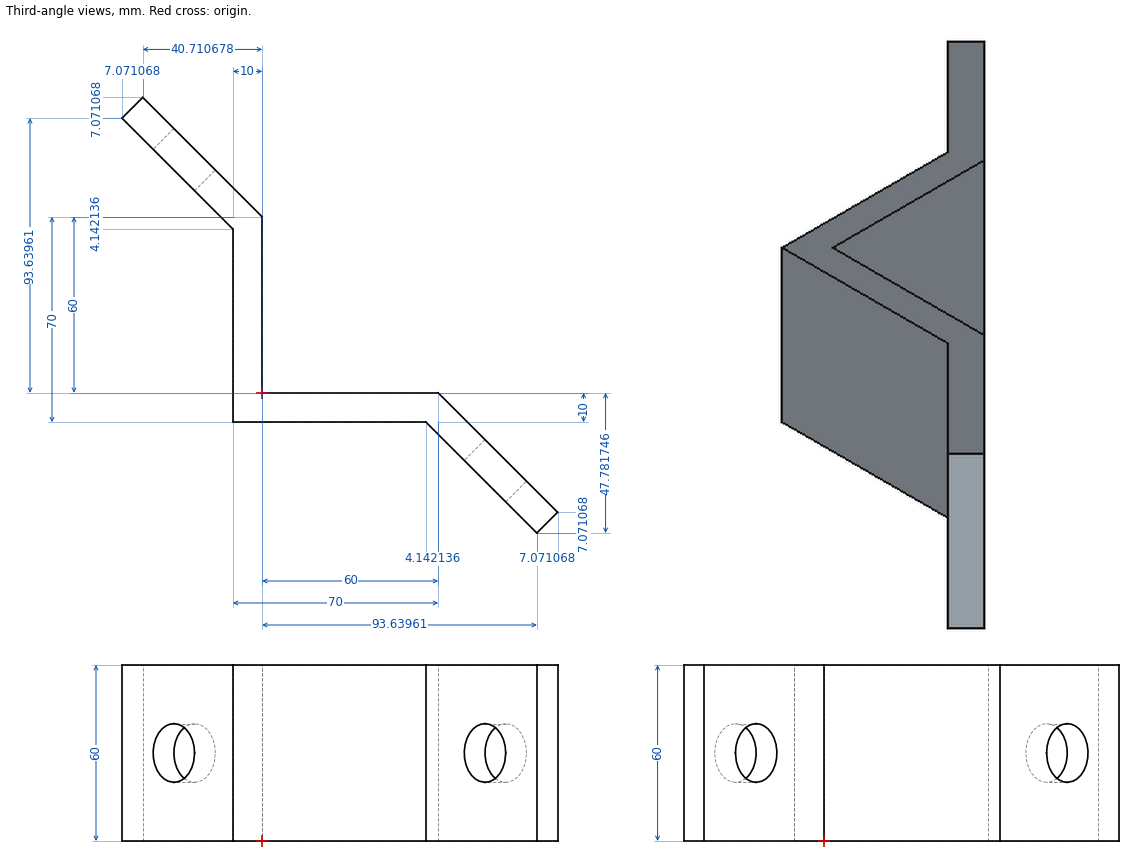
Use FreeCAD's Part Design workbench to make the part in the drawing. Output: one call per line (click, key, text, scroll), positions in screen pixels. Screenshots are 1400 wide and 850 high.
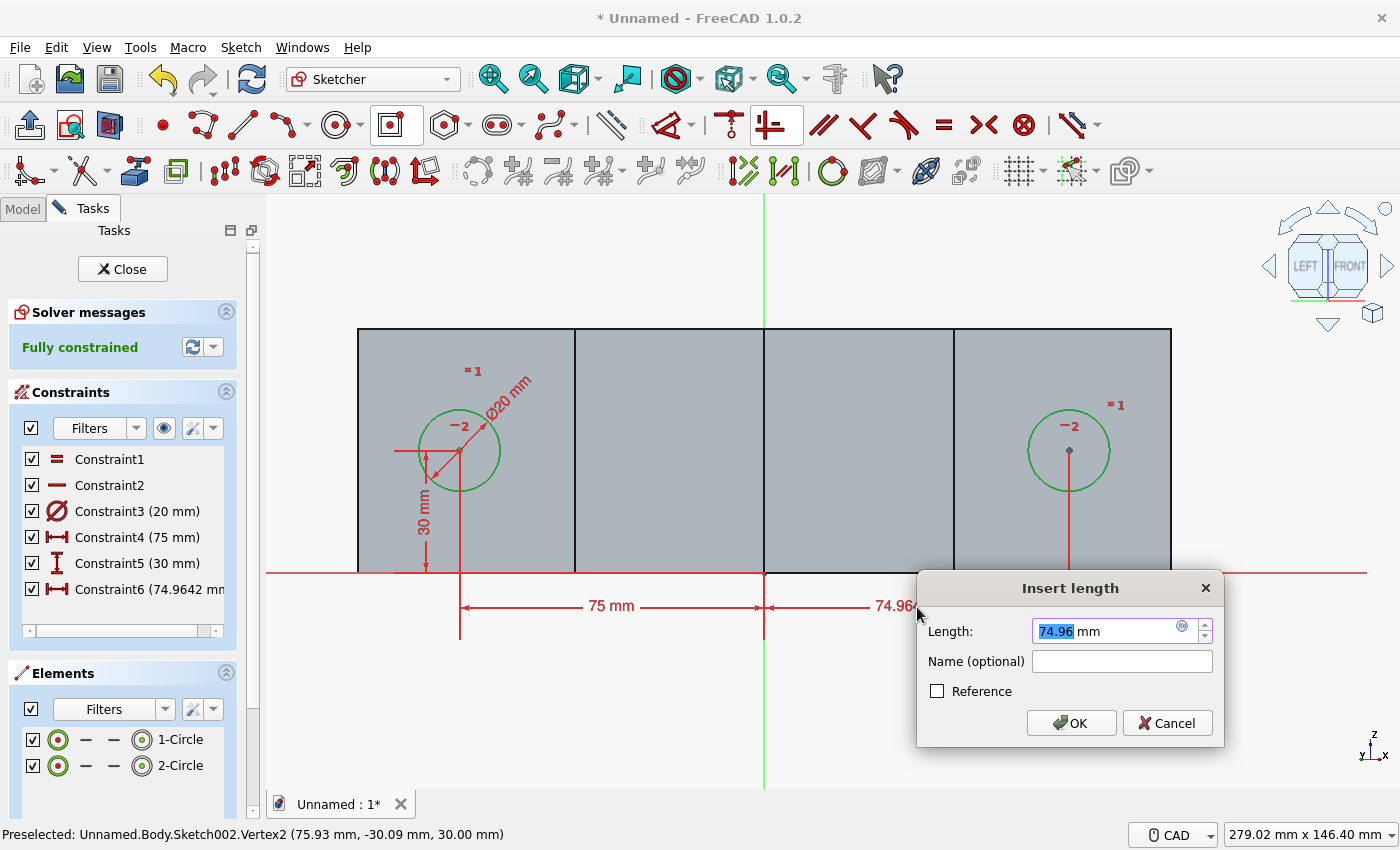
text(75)
key(Return)
key(Escape)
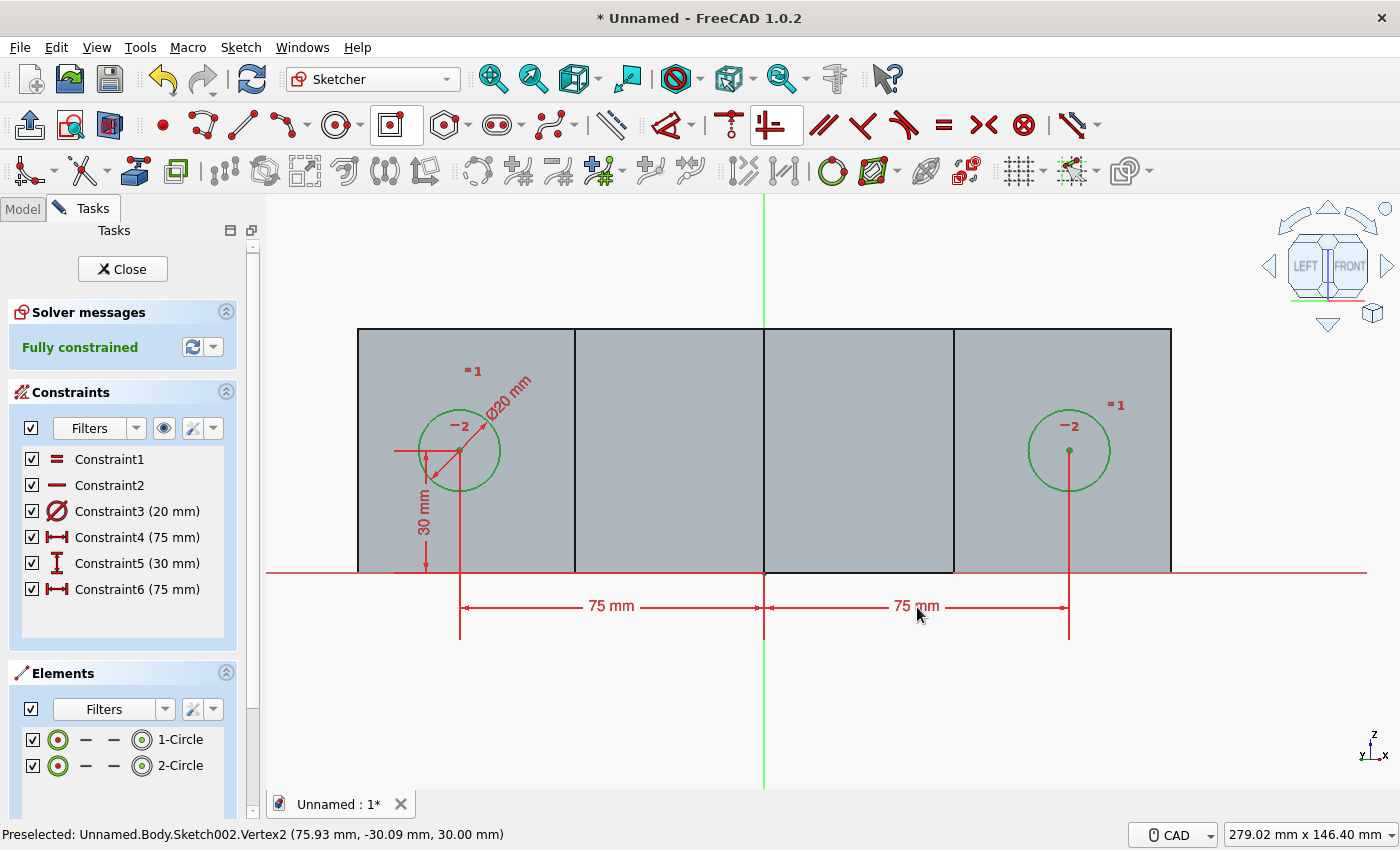
click(123, 269)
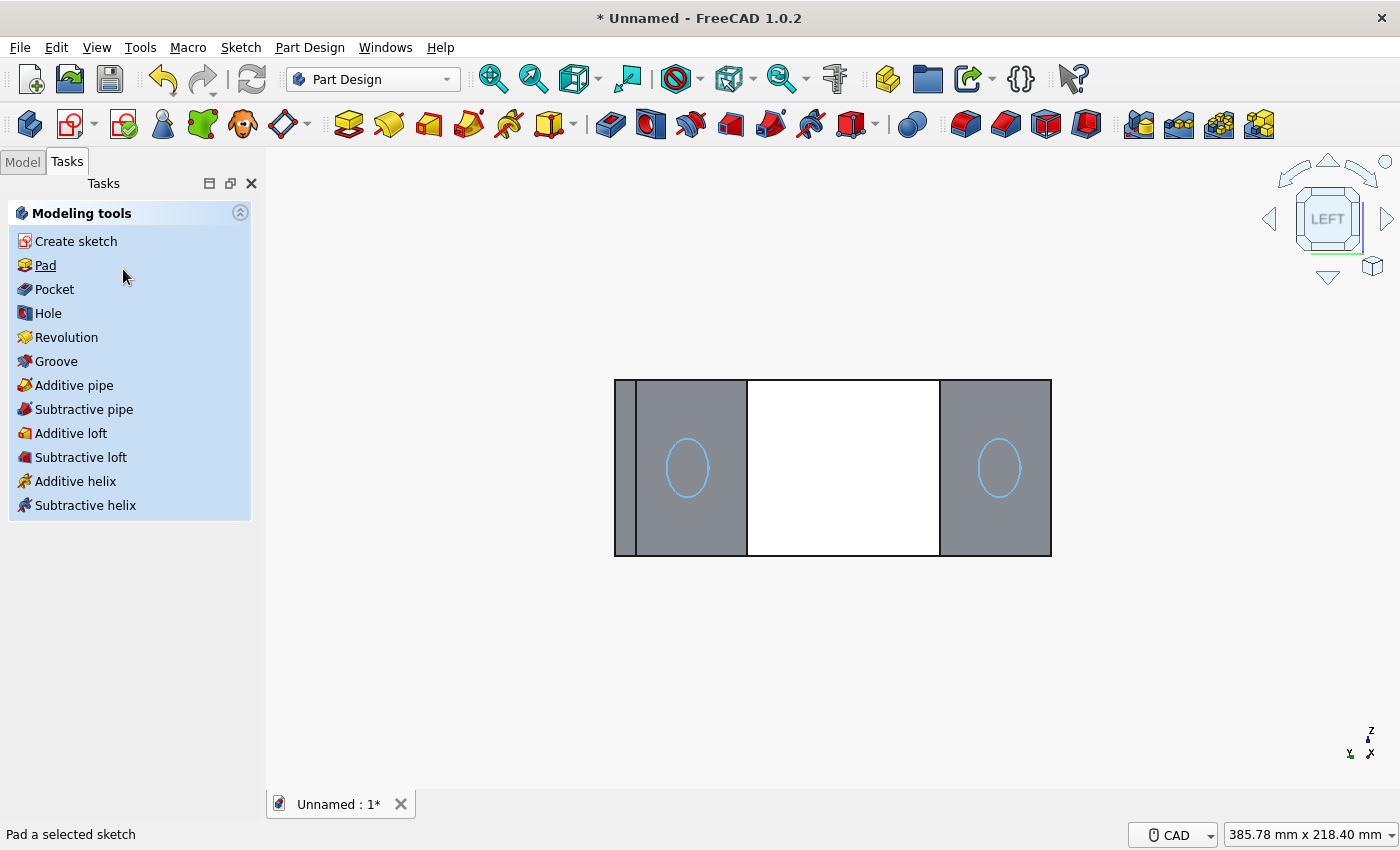
click(612, 124)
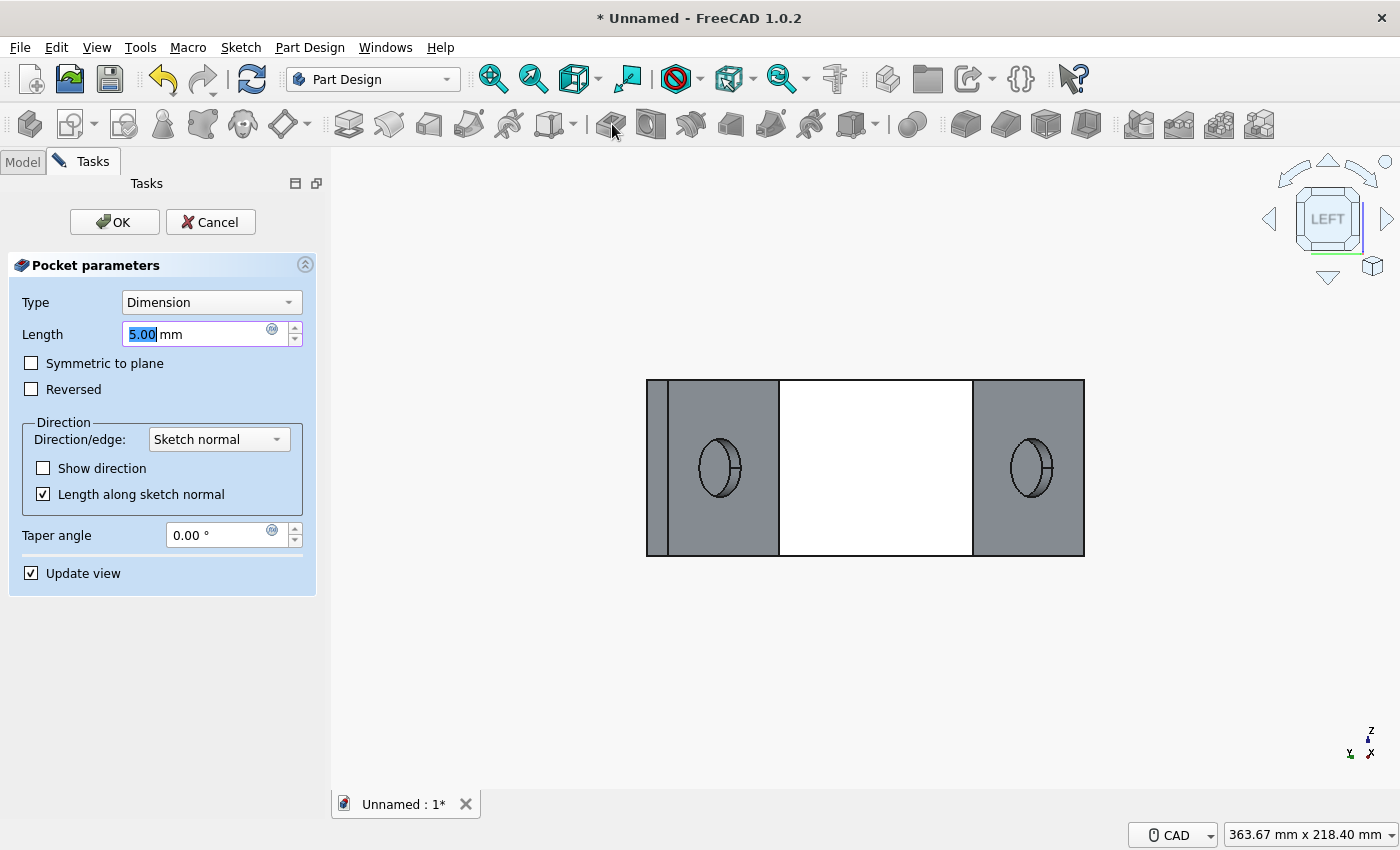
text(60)
key(Tab)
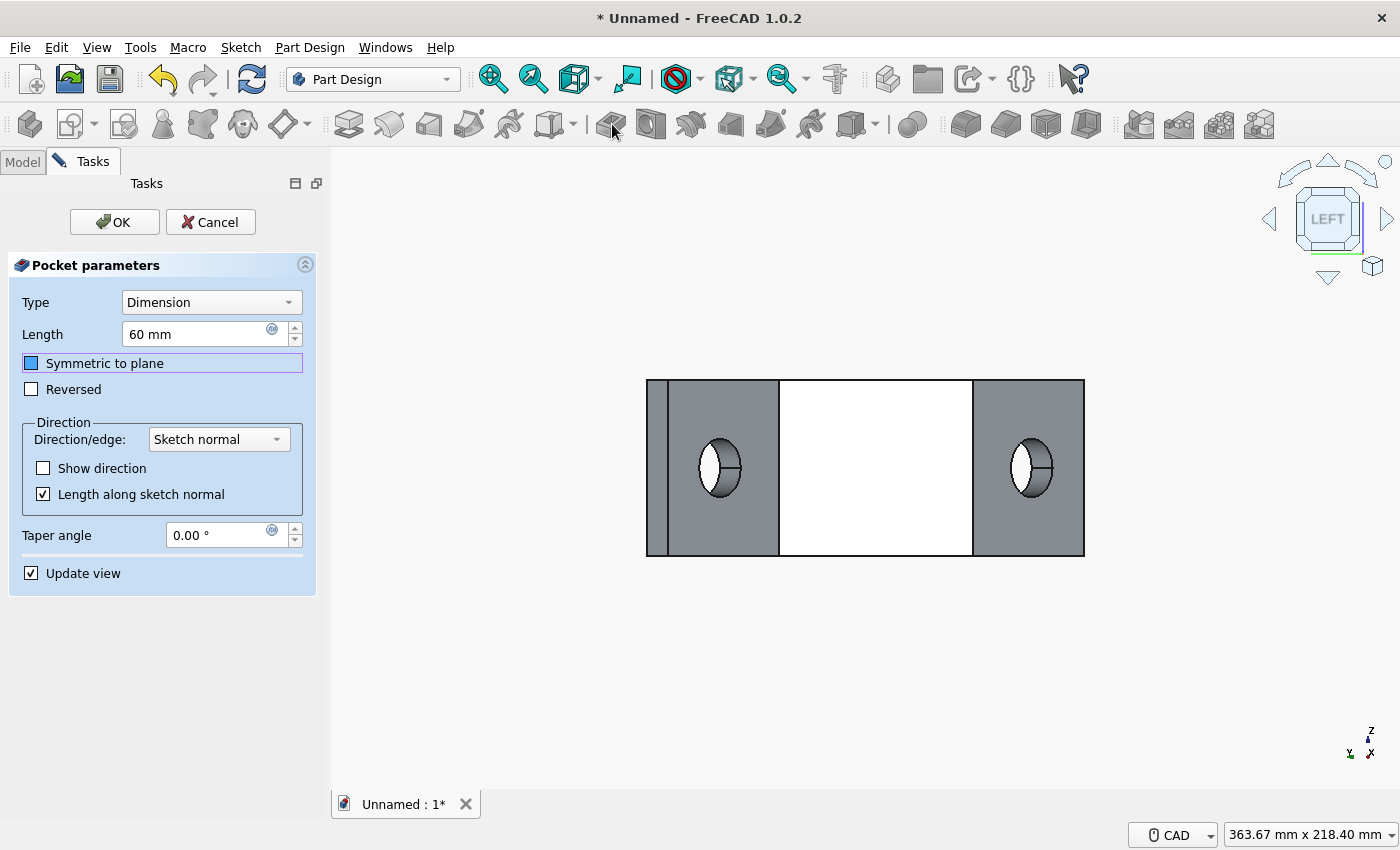
click(115, 222)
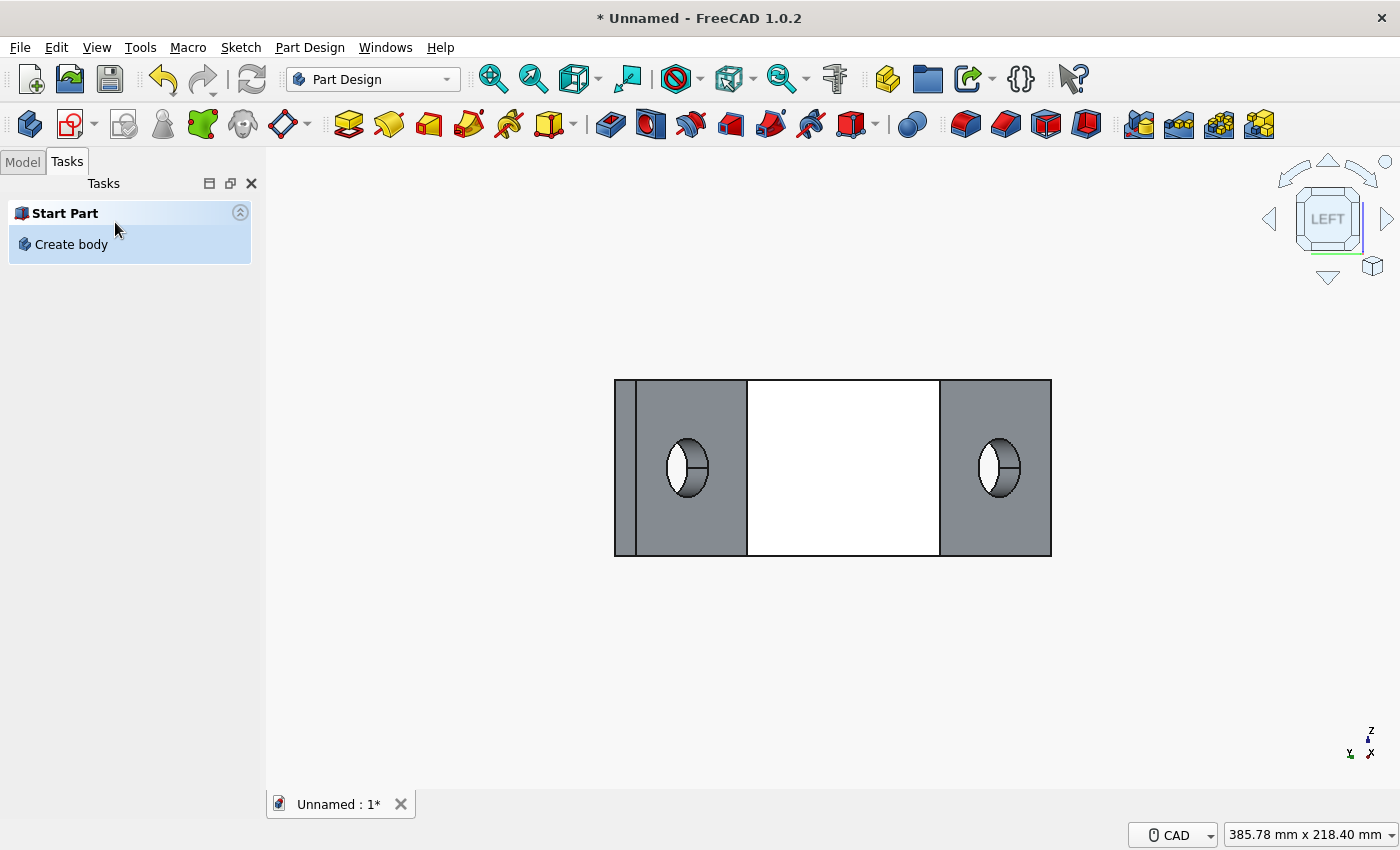
key(0)